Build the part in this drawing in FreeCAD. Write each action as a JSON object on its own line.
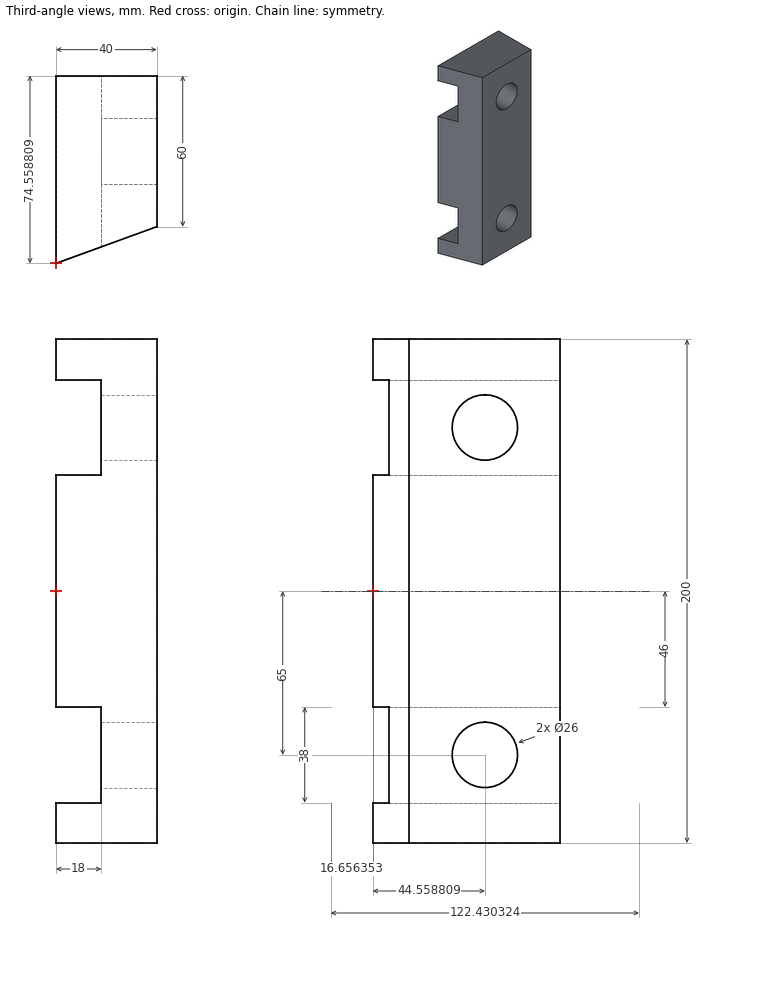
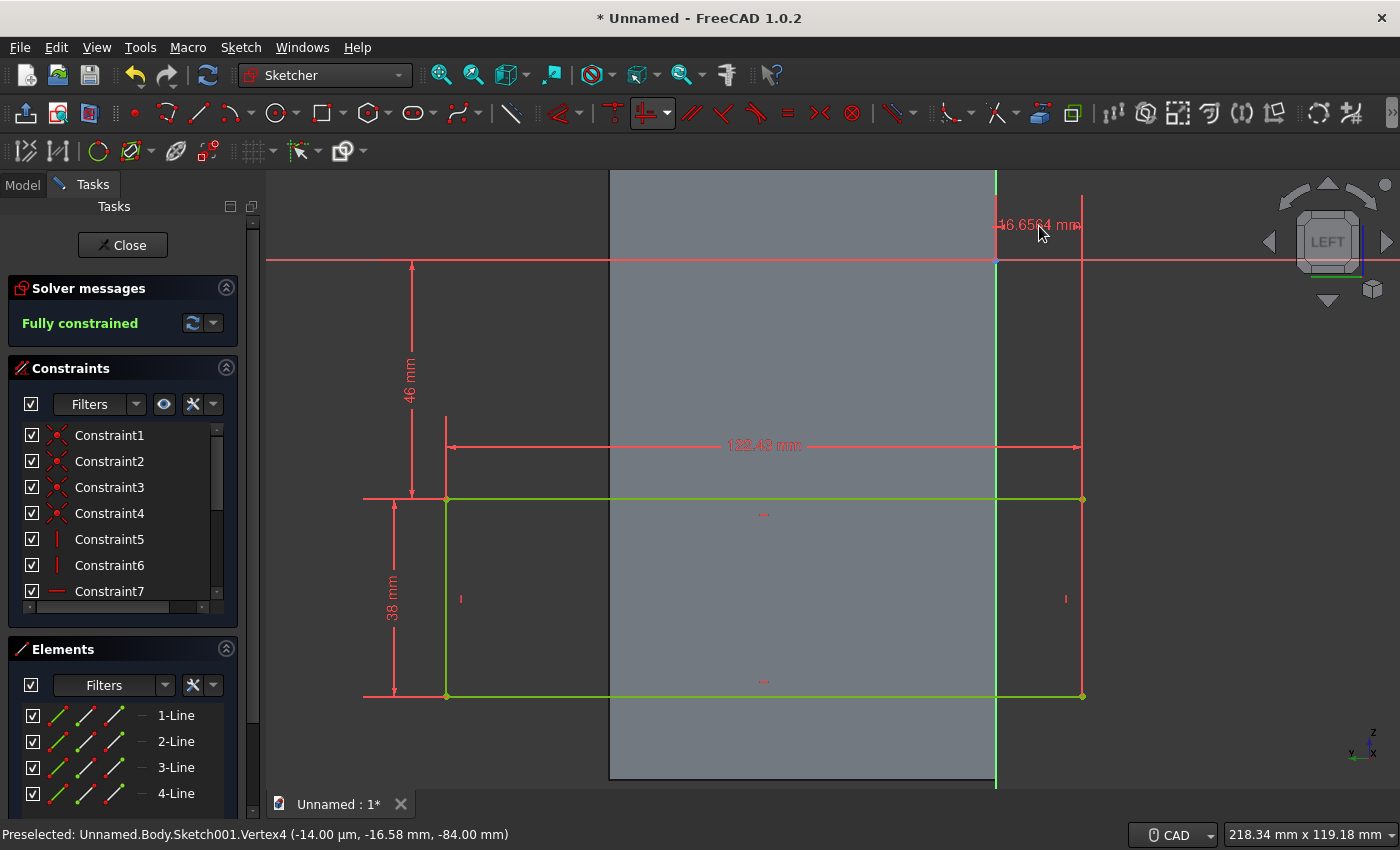
{"action": "left_click", "coordinate": [123, 245]}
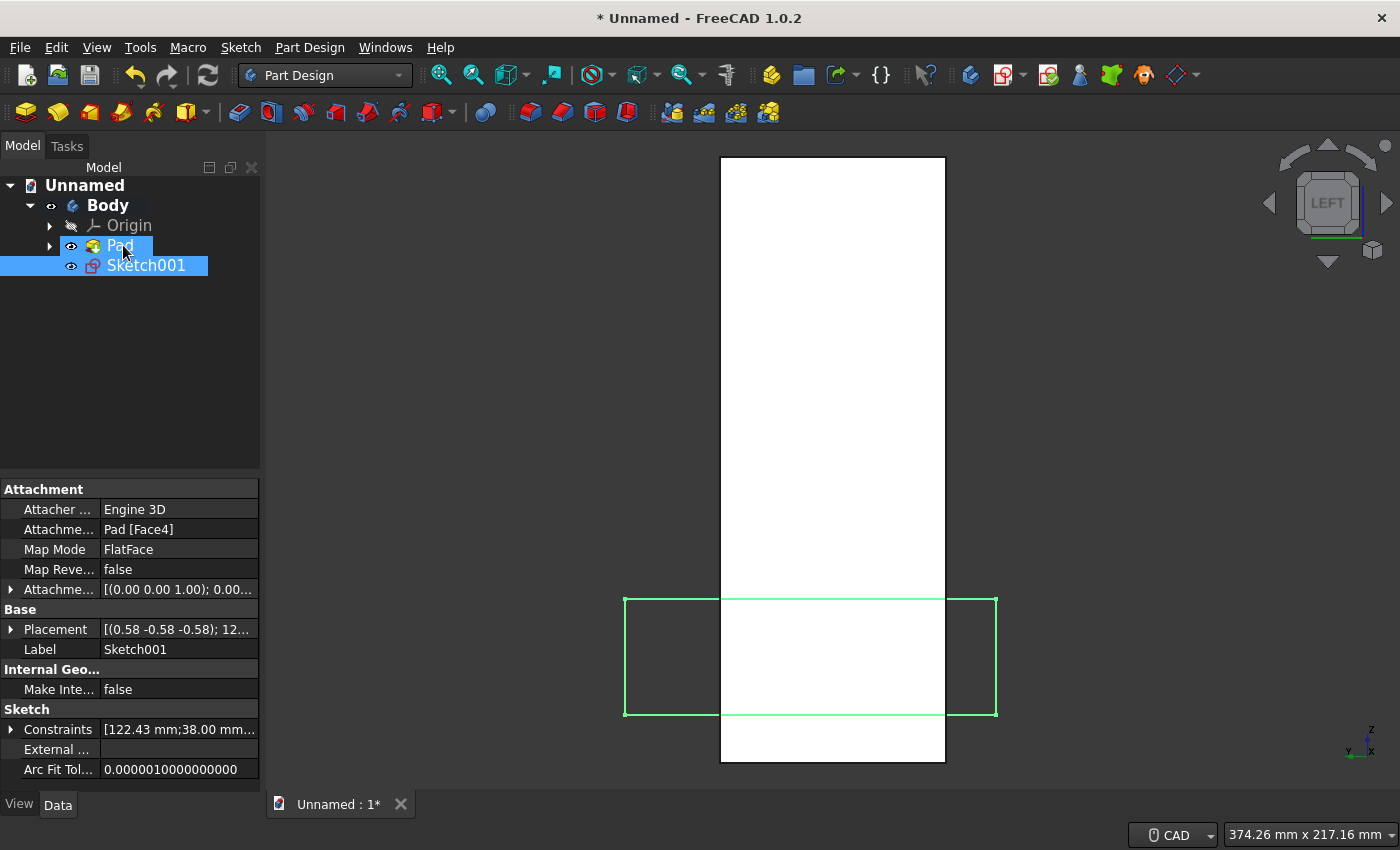
{"action": "left_click", "coordinate": [240, 112]}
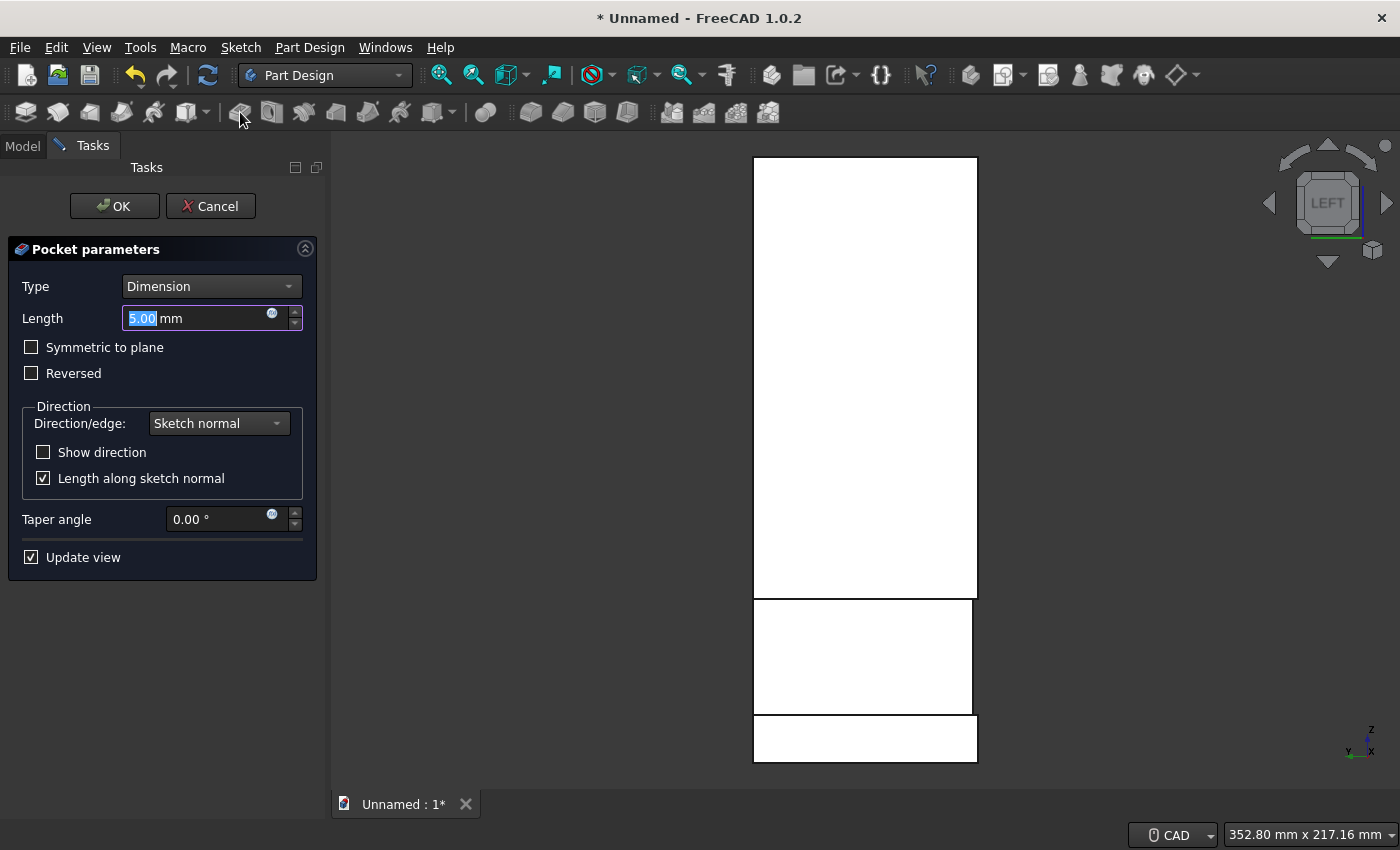
{"action": "type", "text": "18"}
{"action": "key", "text": "Tab"}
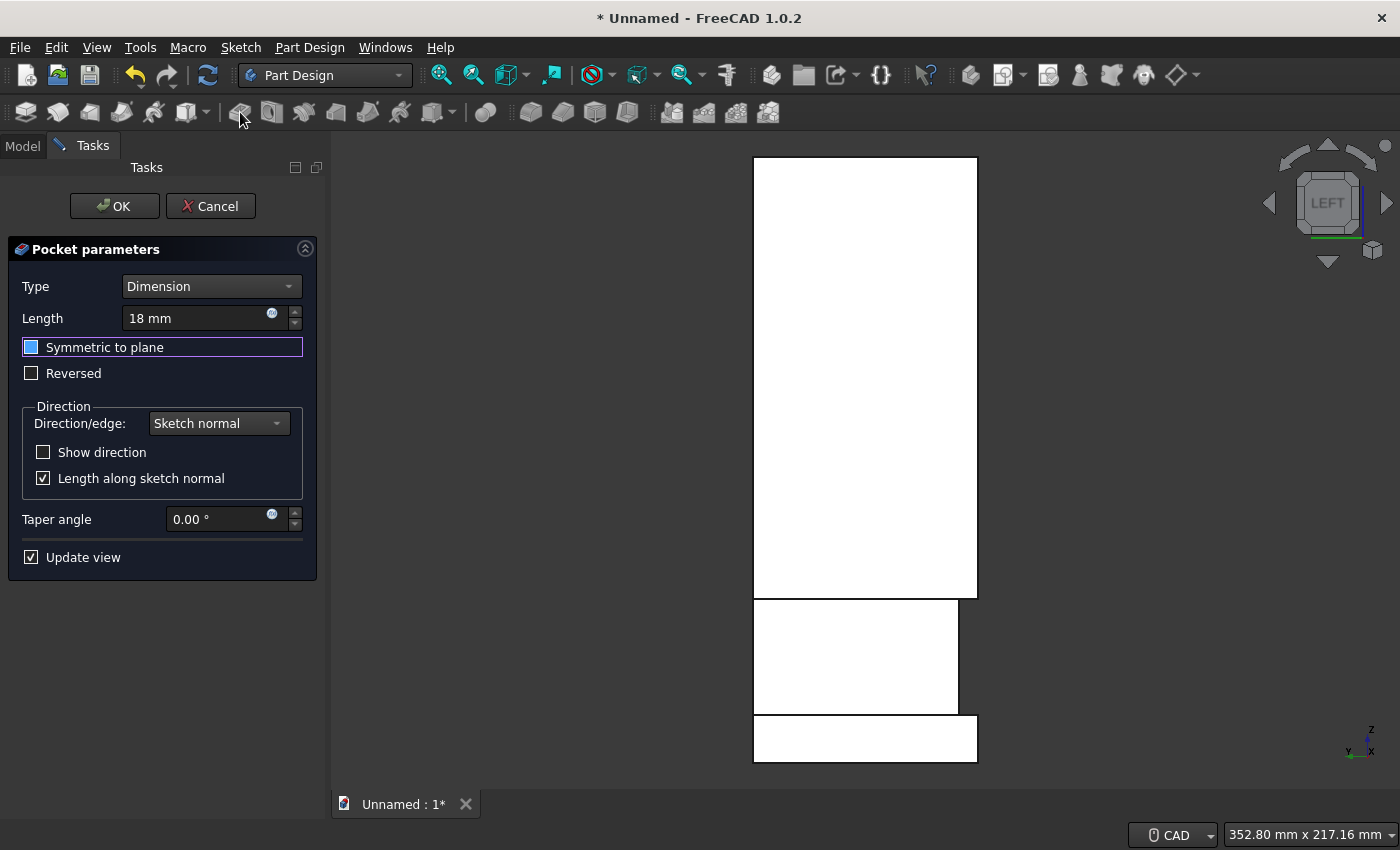
{"action": "left_click", "coordinate": [115, 206]}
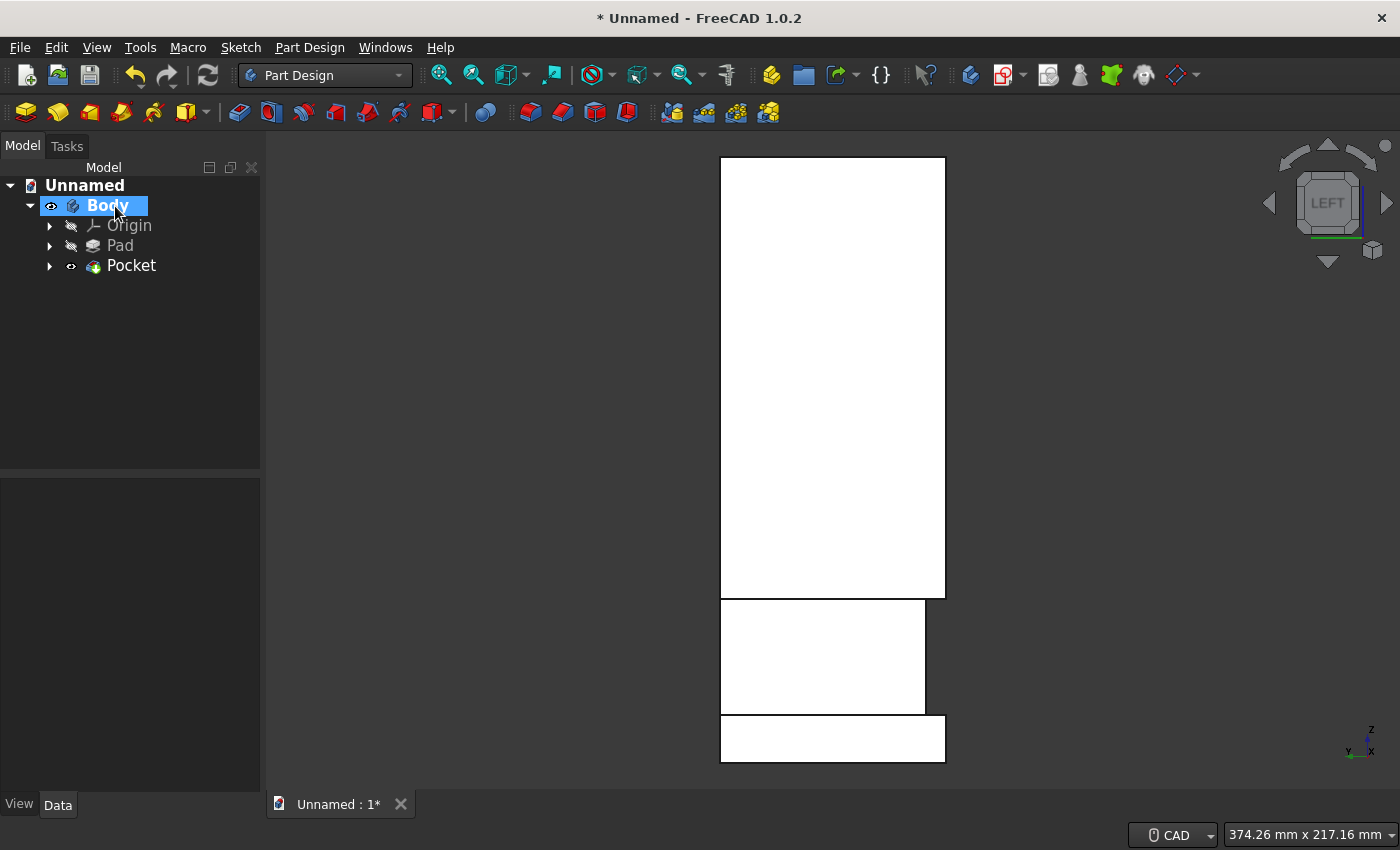
{"action": "left_click", "coordinate": [116, 266]}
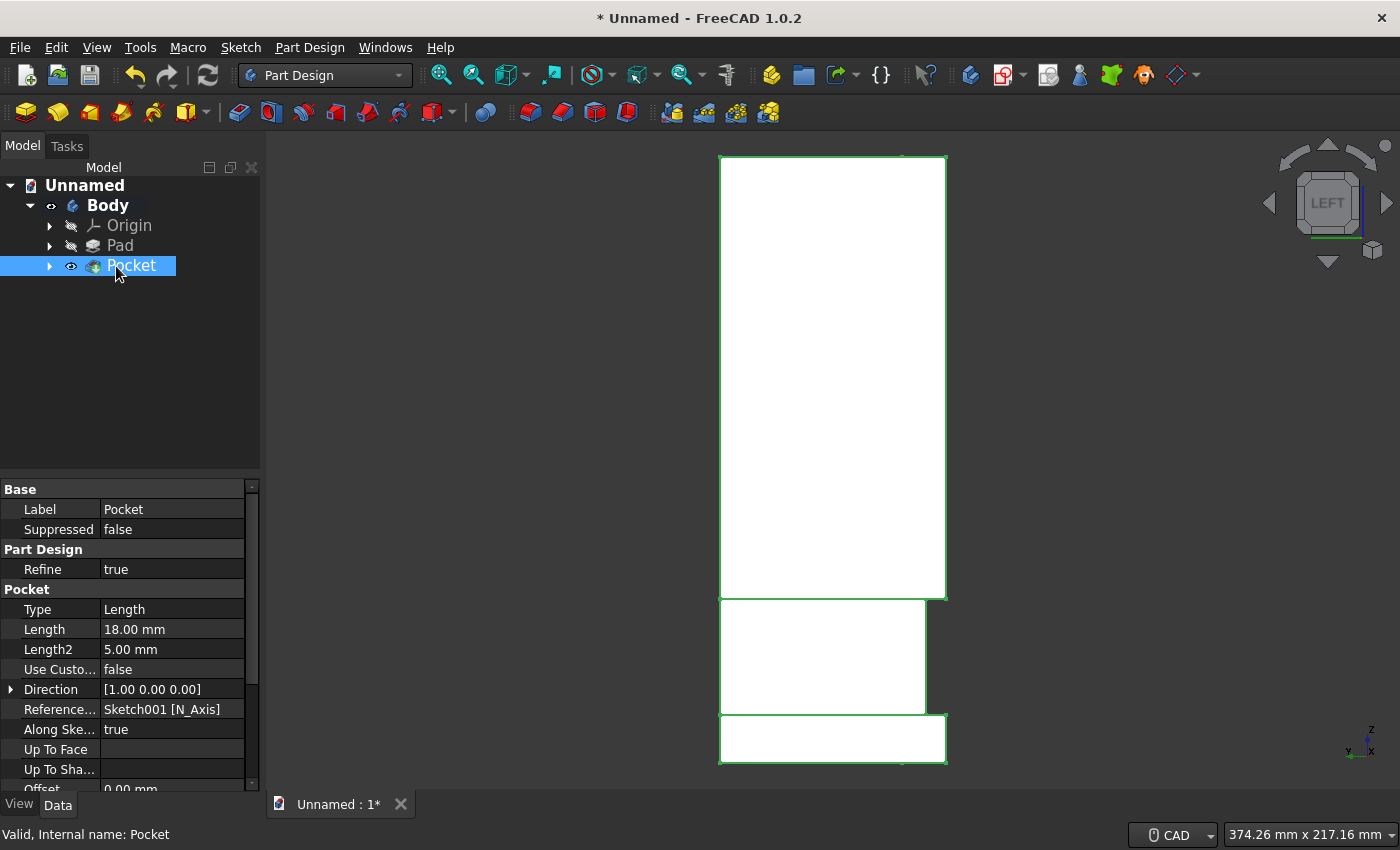
{"action": "left_click", "coordinate": [672, 112]}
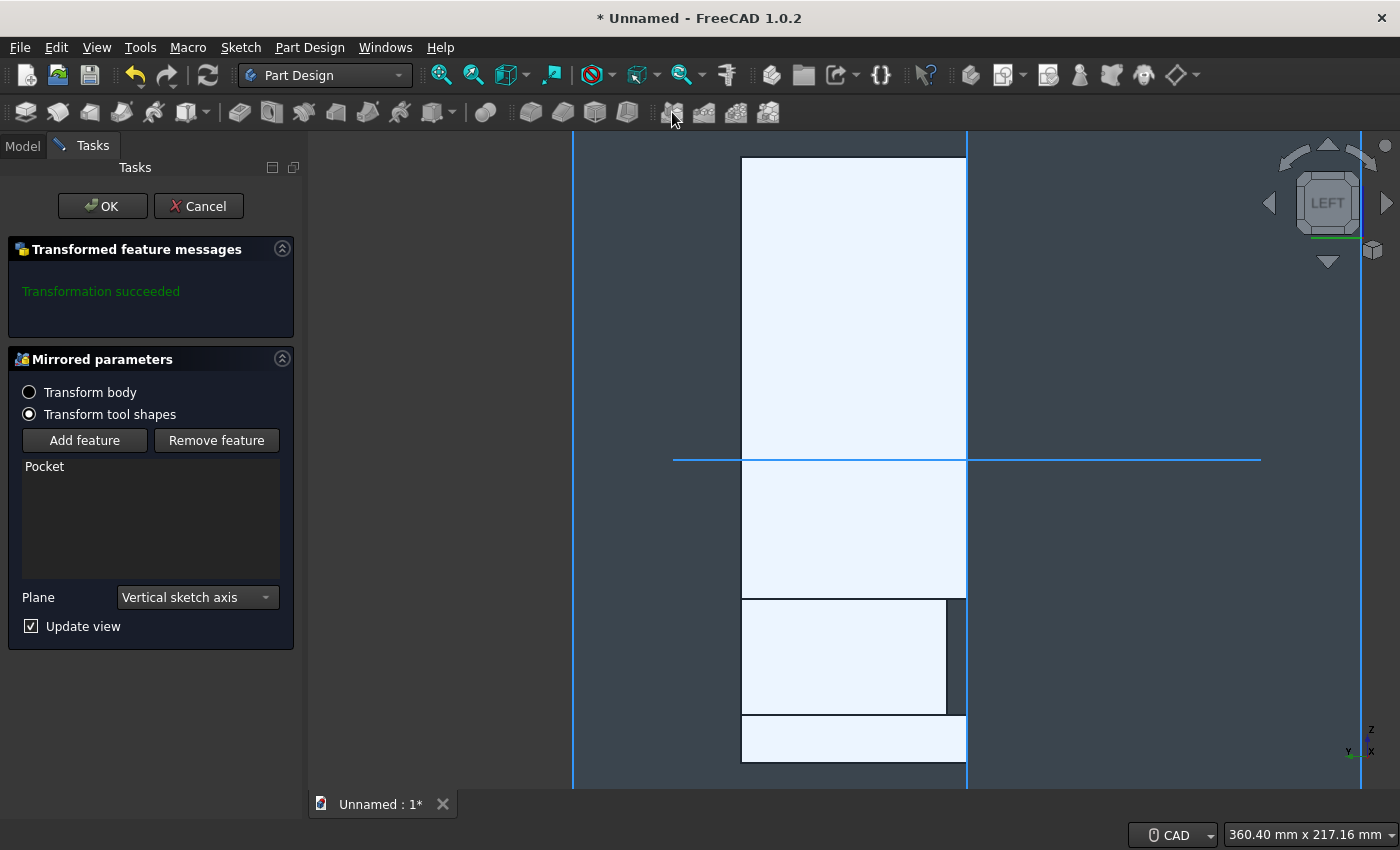
{"action": "left_click", "coordinate": [198, 598]}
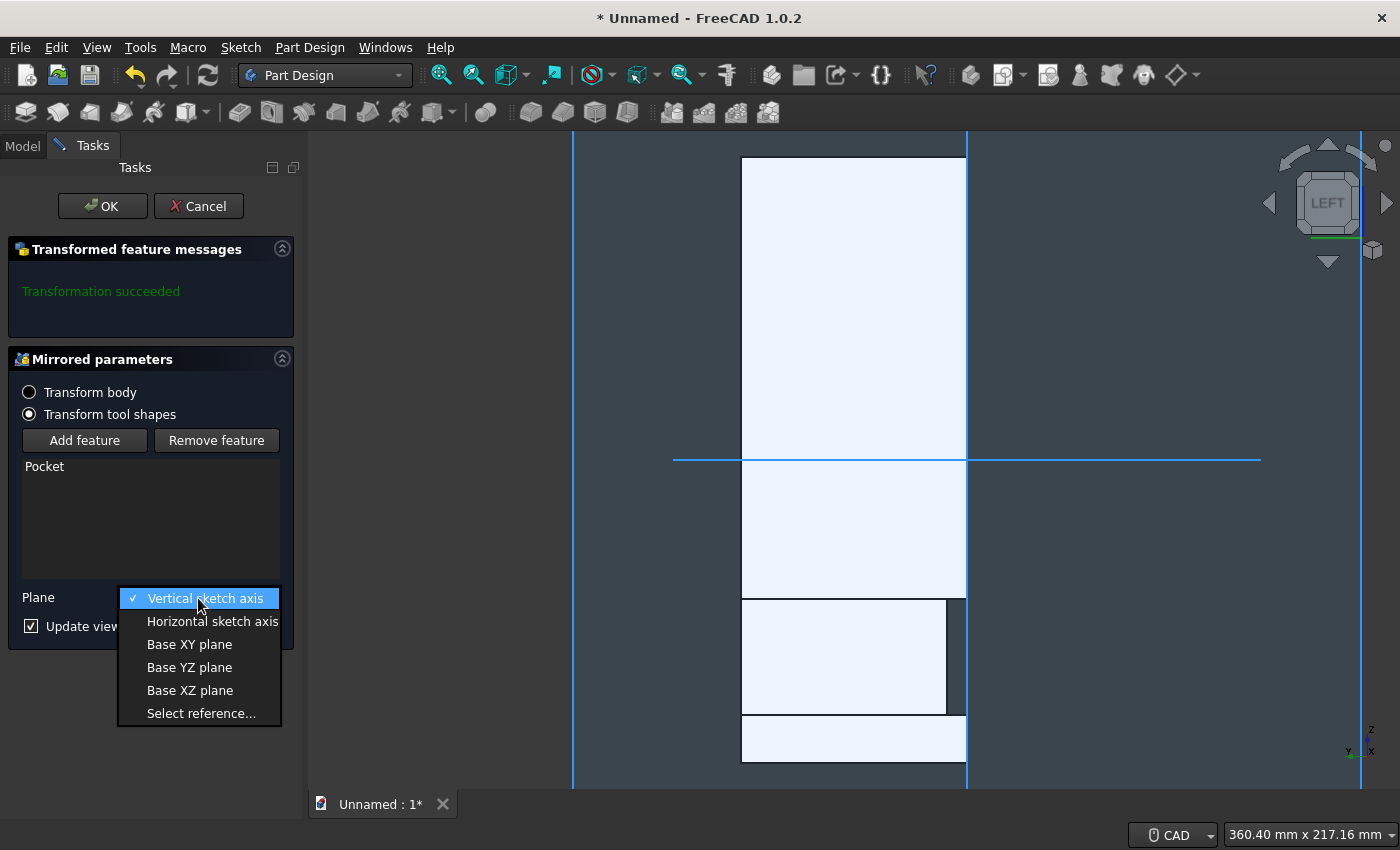
{"action": "left_click", "coordinate": [198, 644]}